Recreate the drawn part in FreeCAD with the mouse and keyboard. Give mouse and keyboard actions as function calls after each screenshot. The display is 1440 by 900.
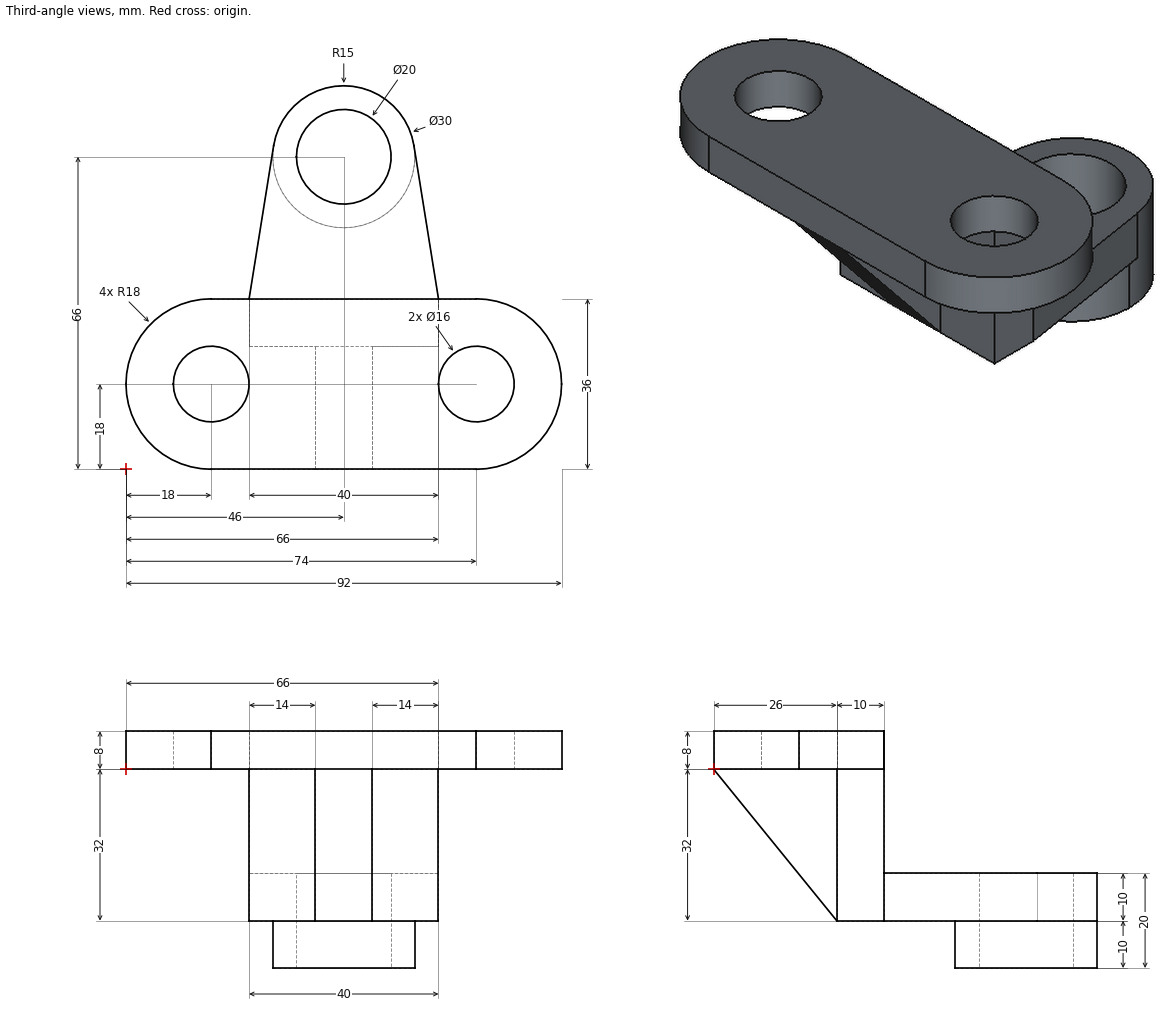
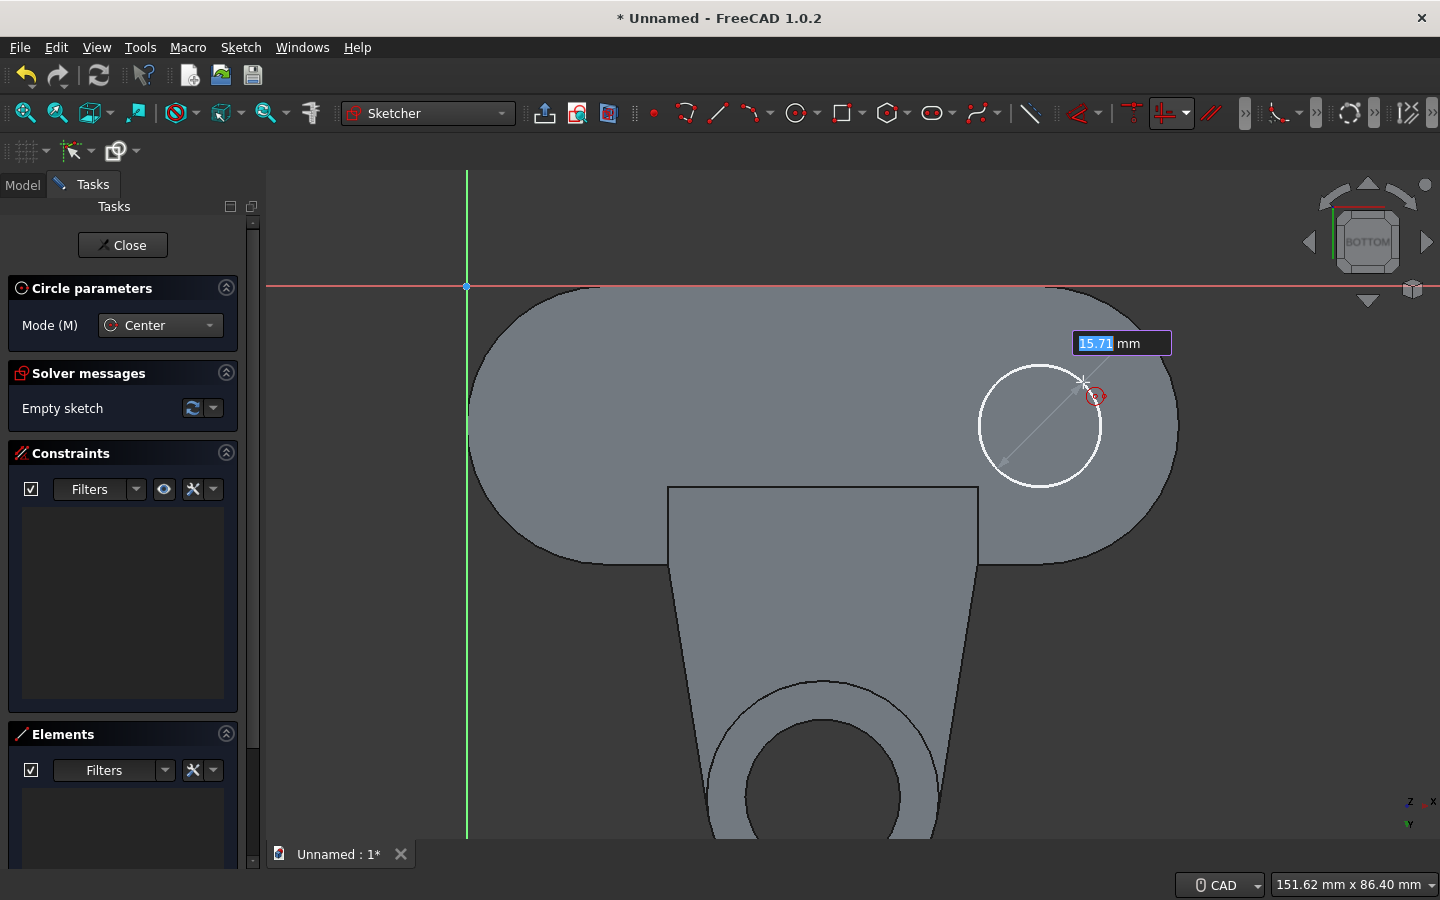
text(16)
key(Return)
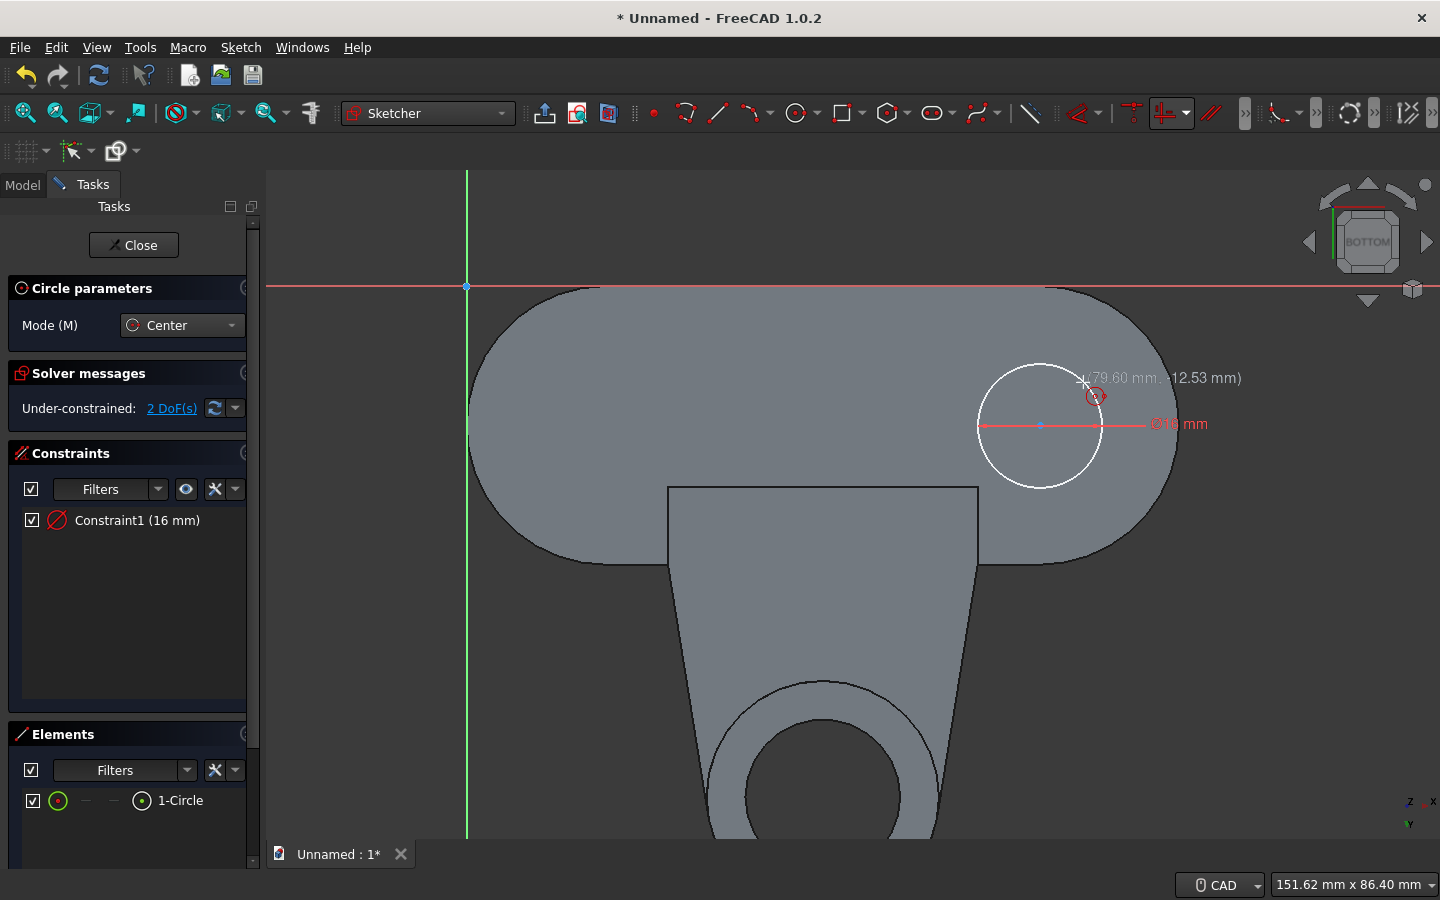
click(606, 425)
move(650, 382)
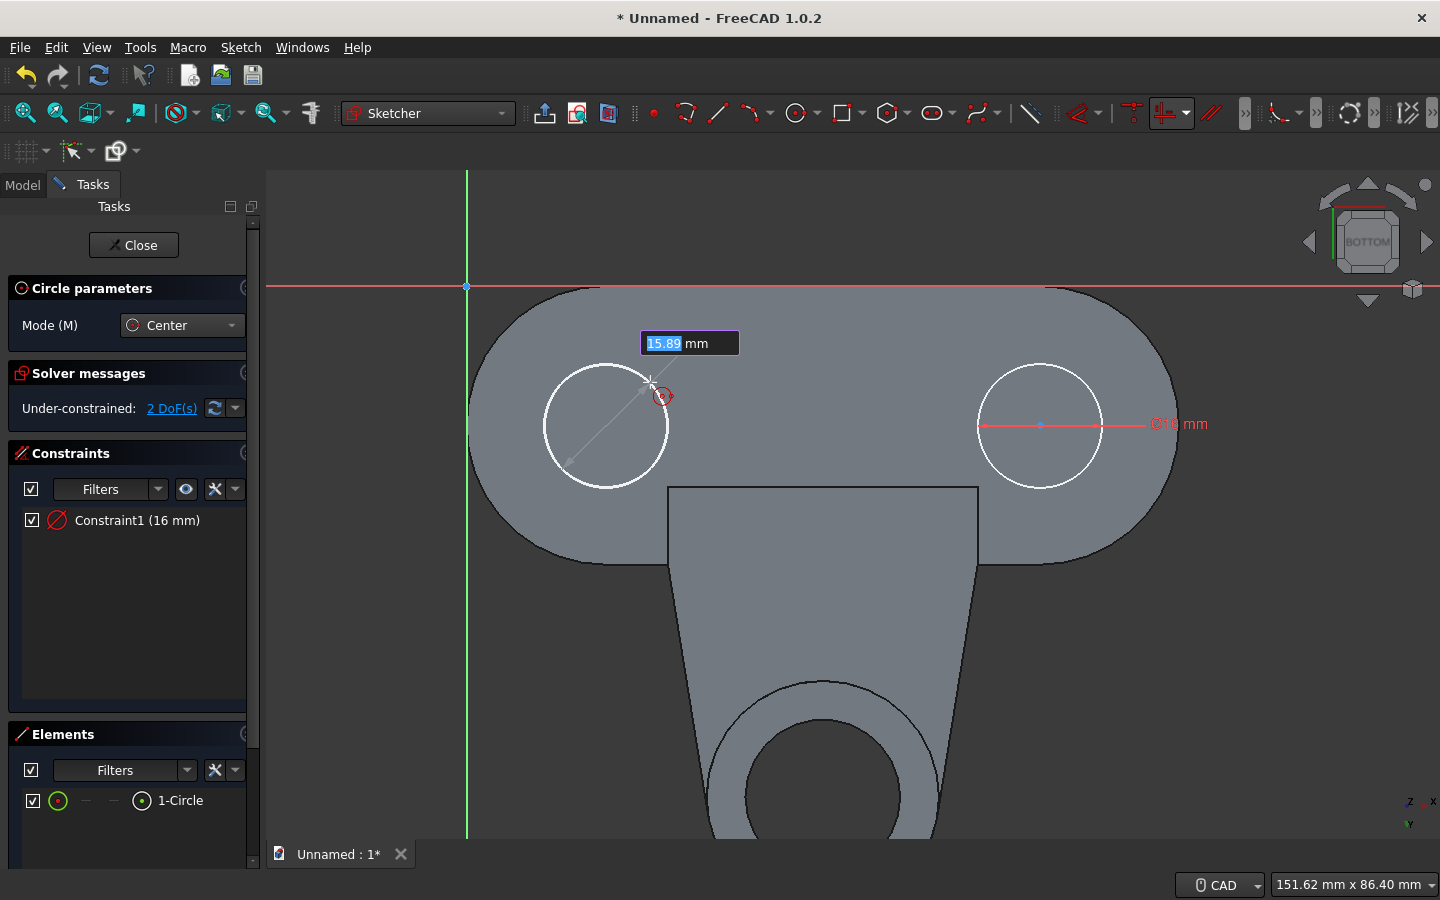
text(16)
key(Return)
key(Escape)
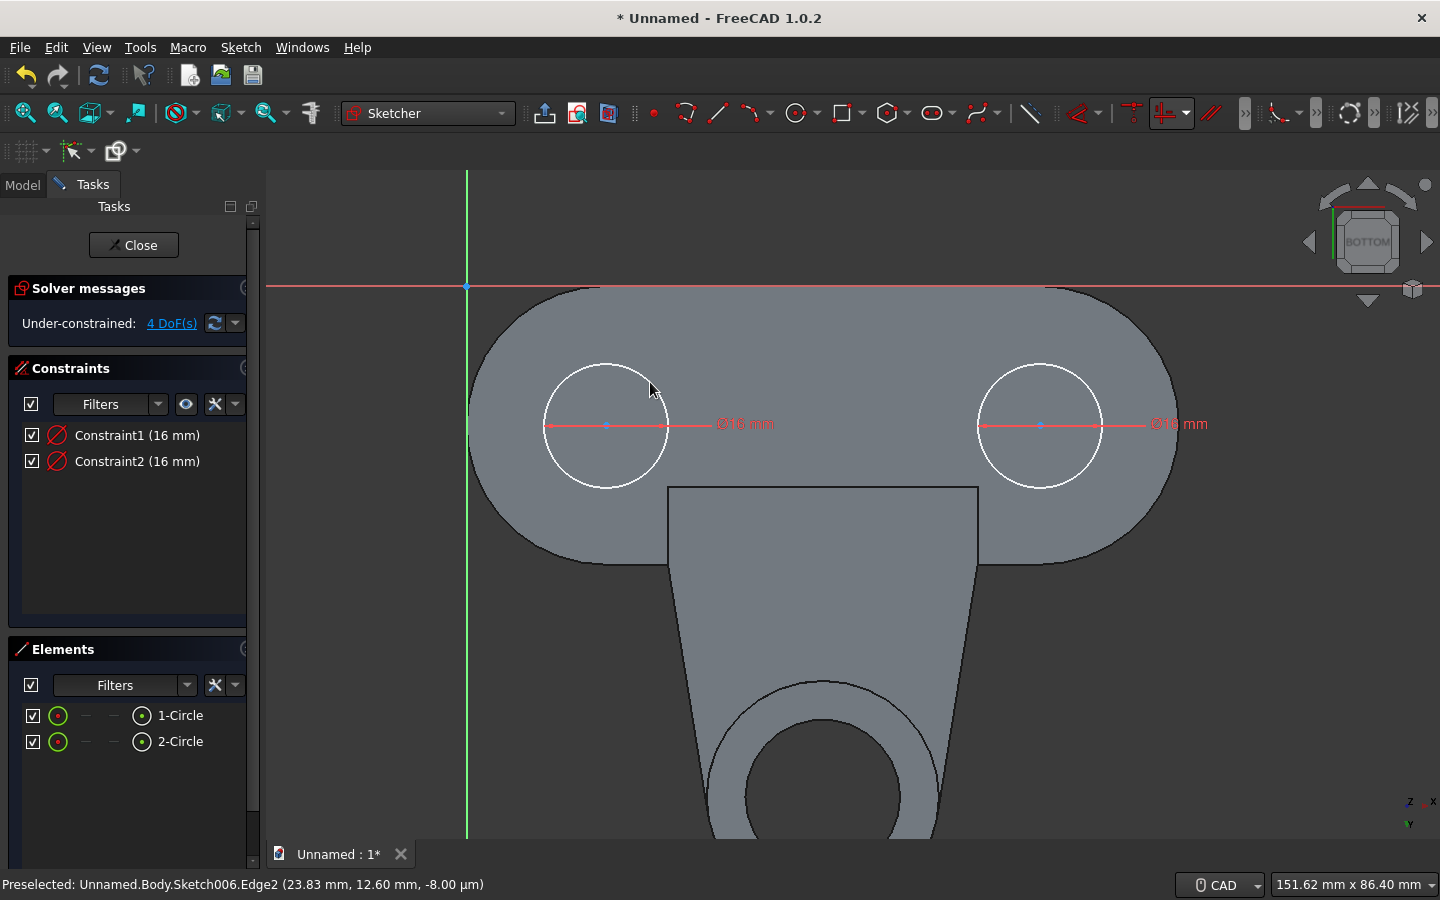
click(1040, 426)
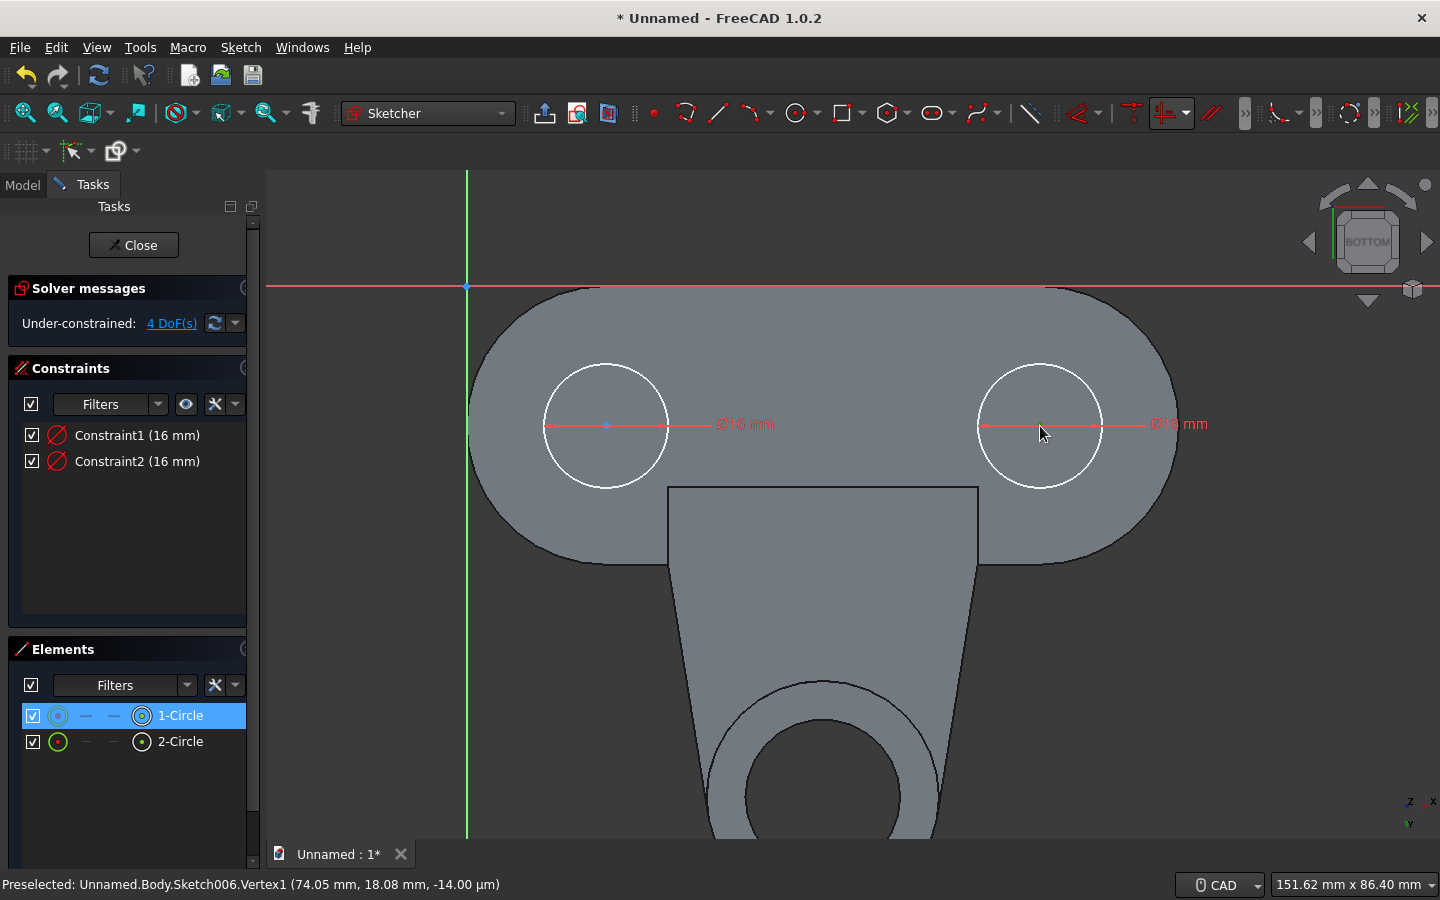
click(606, 426)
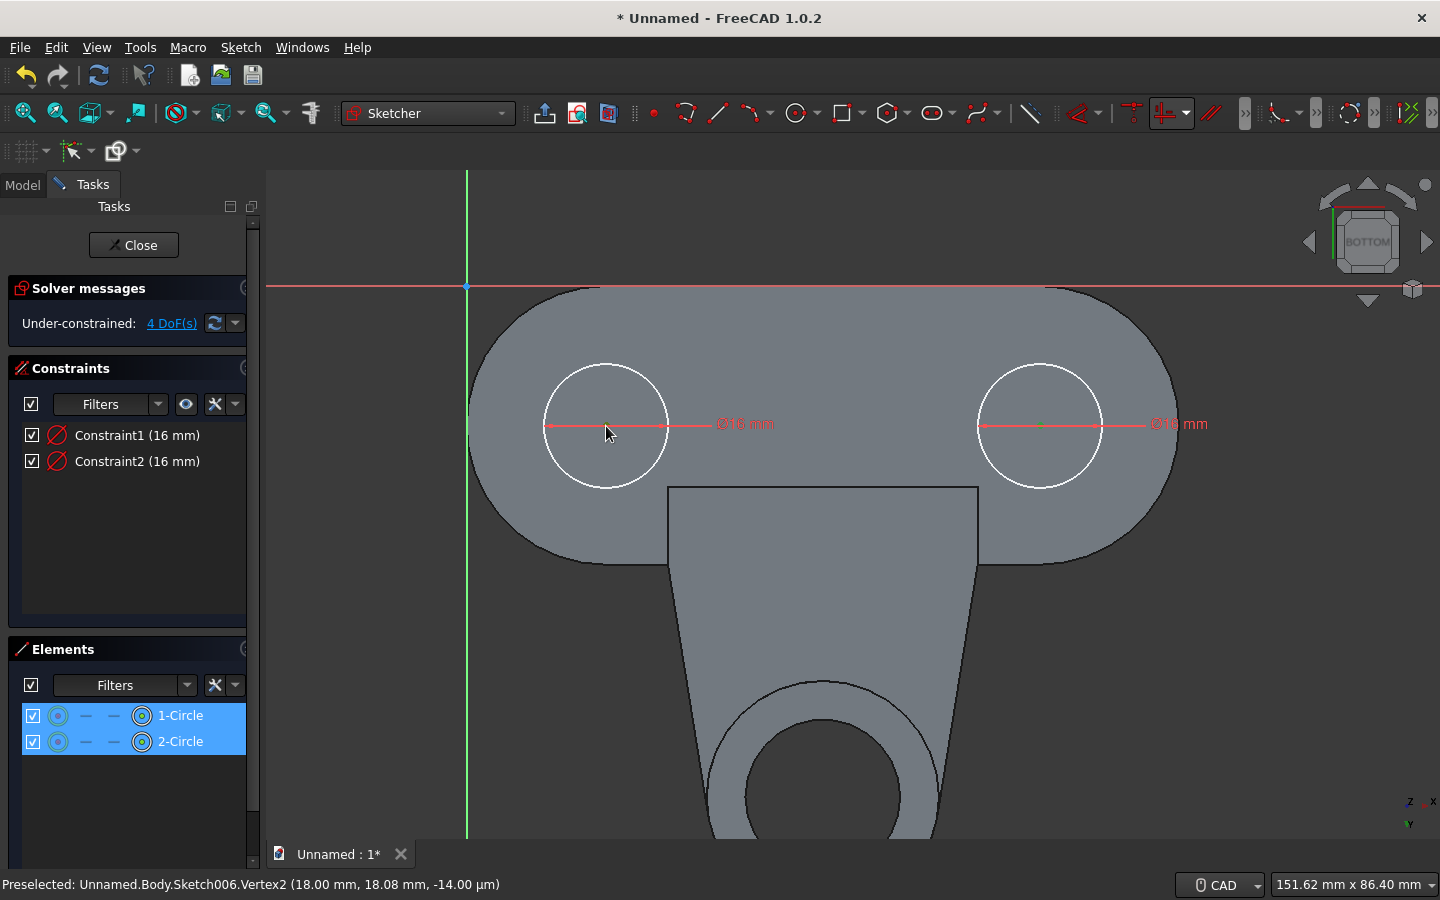
key(h)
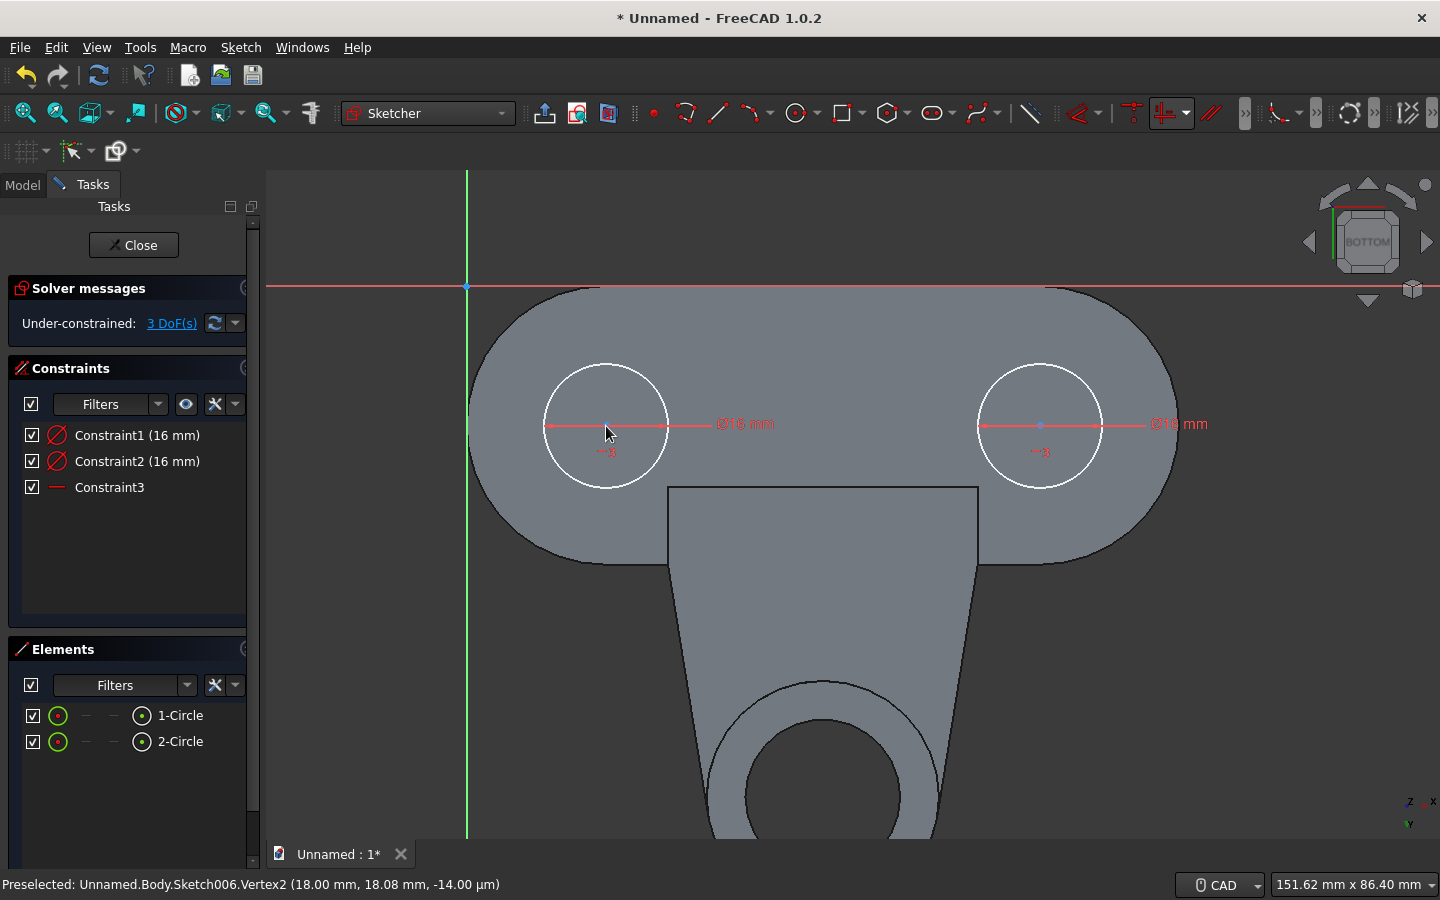
click(1078, 114)